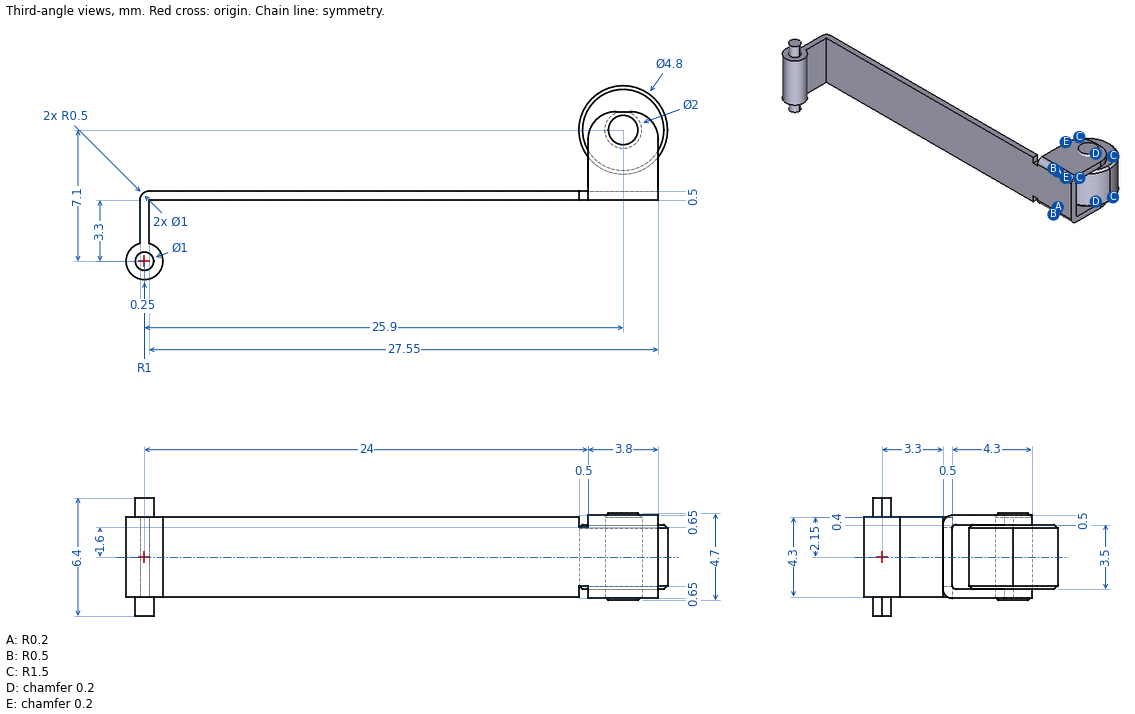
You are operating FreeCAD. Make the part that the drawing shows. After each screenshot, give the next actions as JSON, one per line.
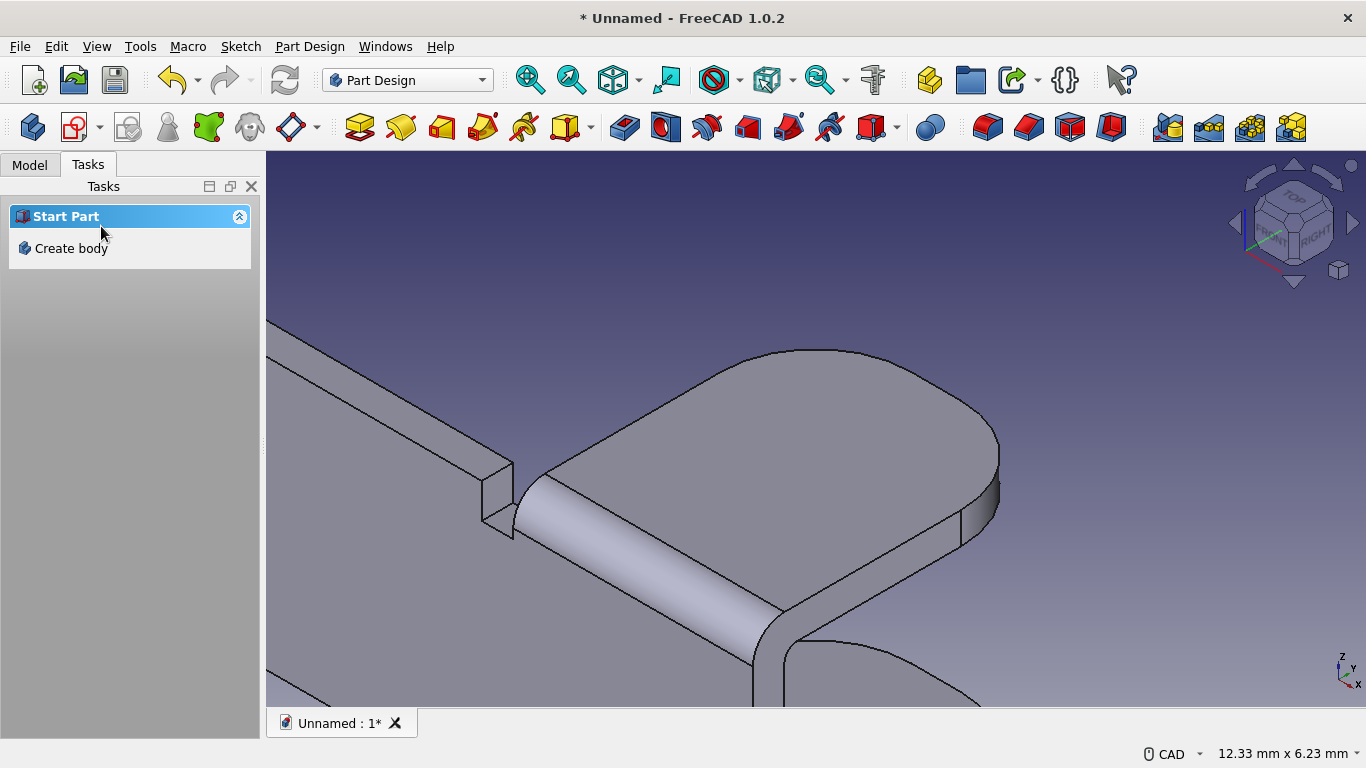
{"action": "left_click", "coordinate": [531, 80]}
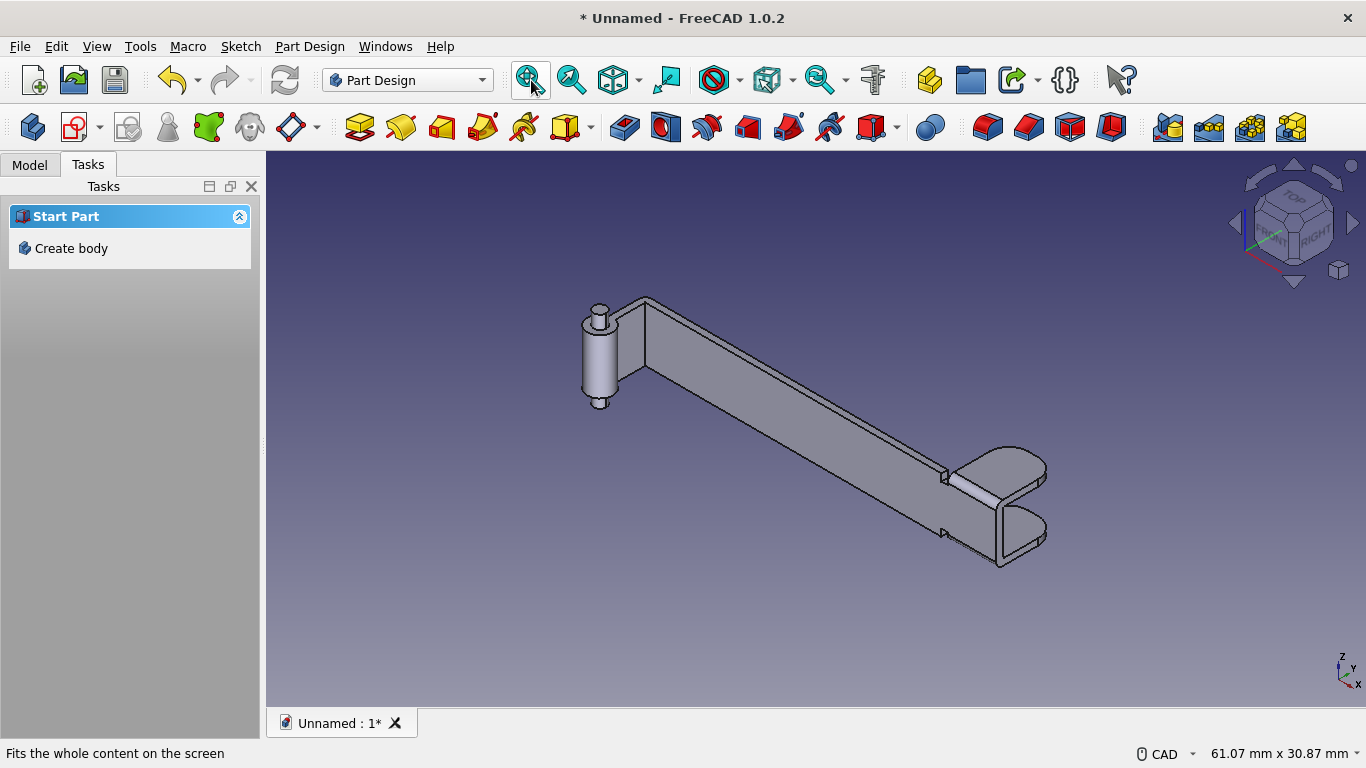
{"action": "left_click", "coordinate": [33, 128]}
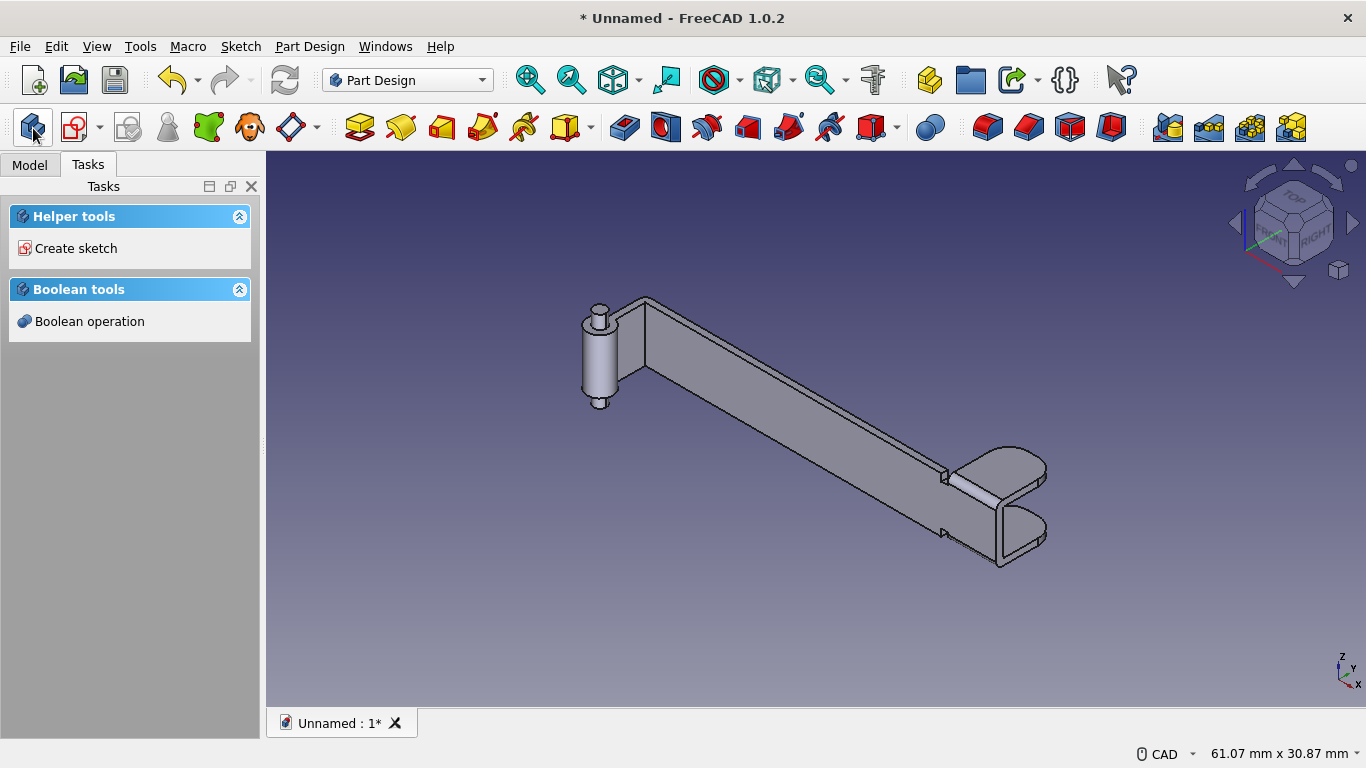
{"action": "left_click", "coordinate": [306, 667]}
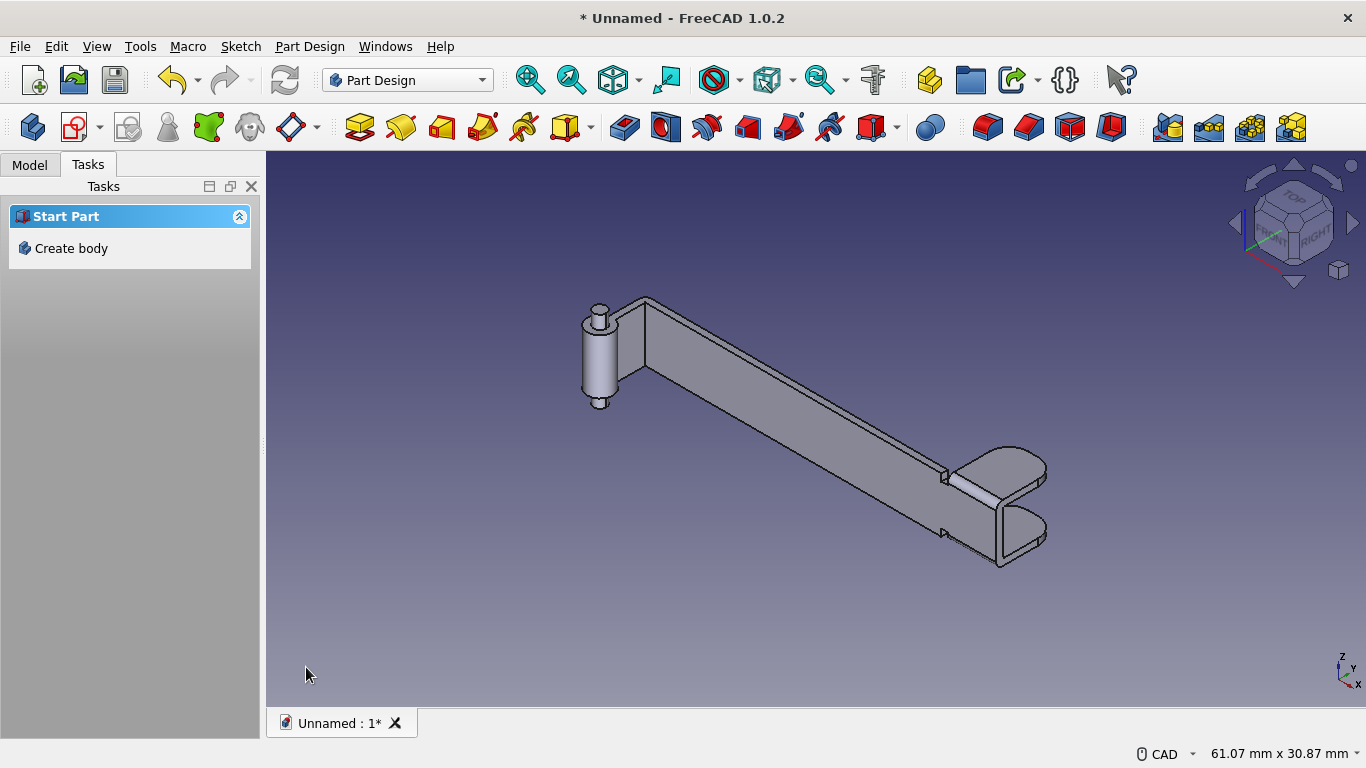
{"action": "left_click", "coordinate": [74, 128]}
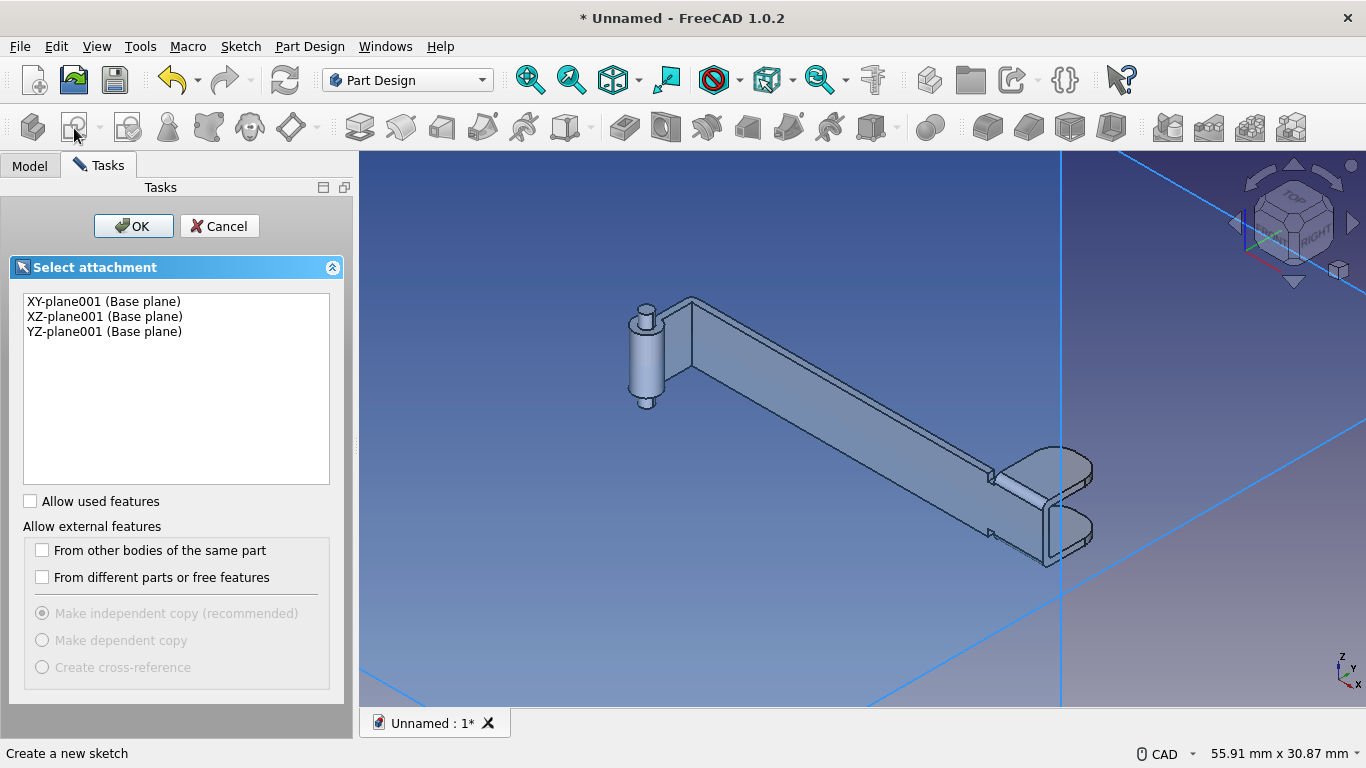
{"action": "left_click", "coordinate": [84, 302]}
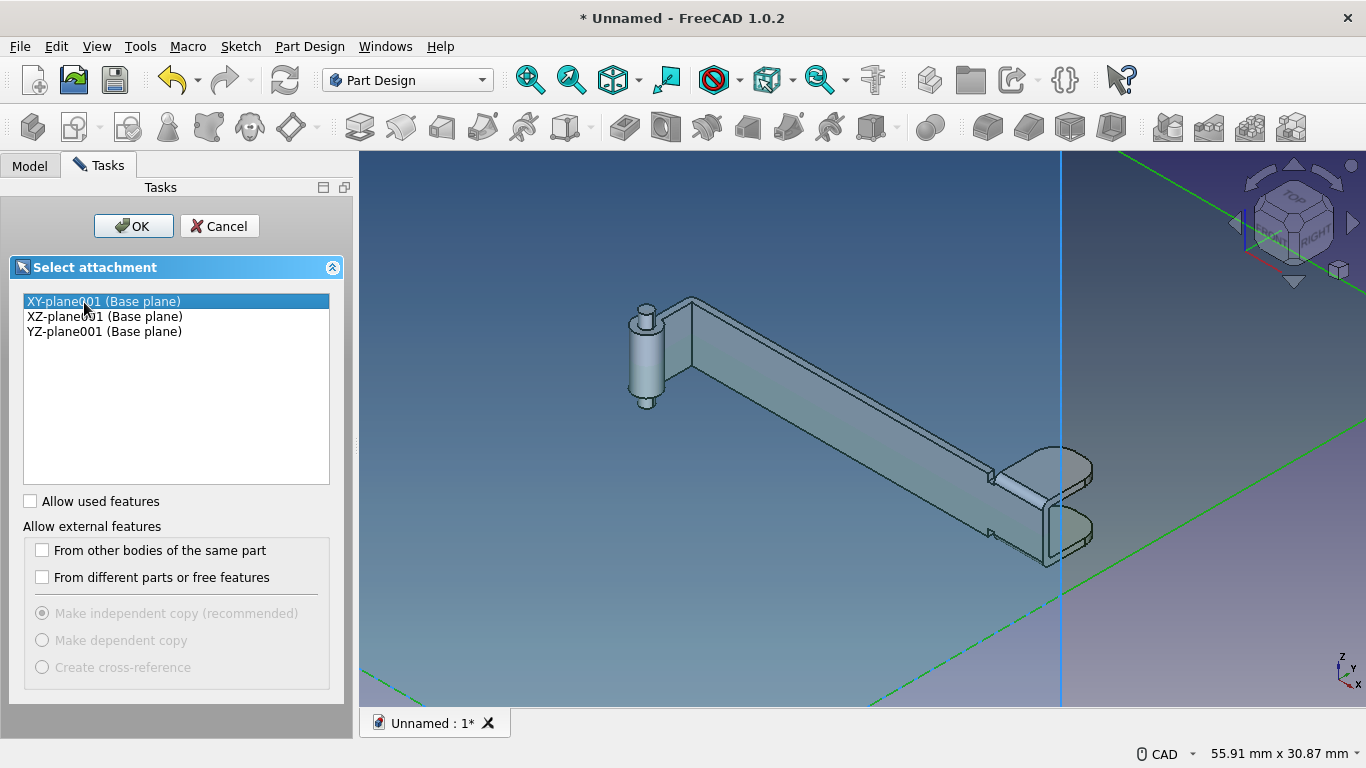
{"action": "left_click", "coordinate": [134, 226]}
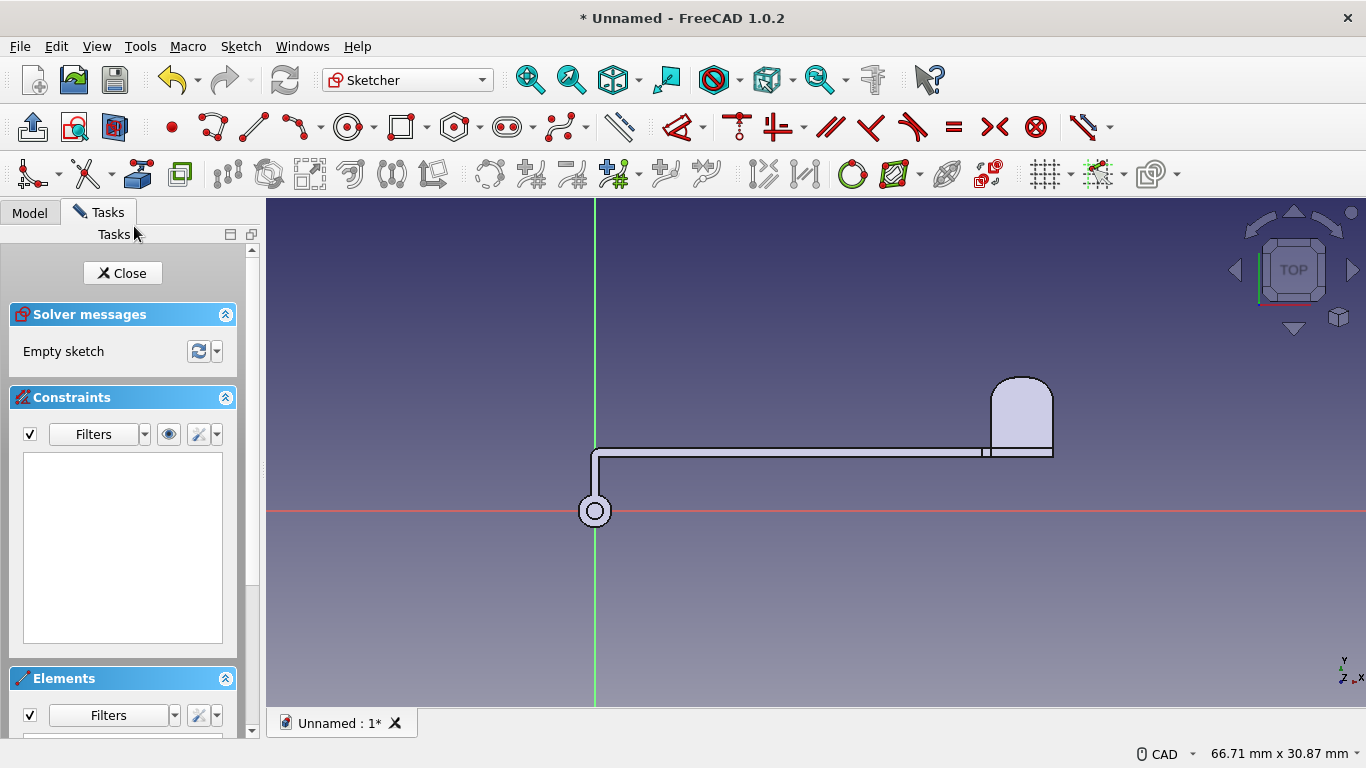
{"action": "scroll", "coordinate": [1056, 387], "scroll_direction": "up", "scroll_amount": 11}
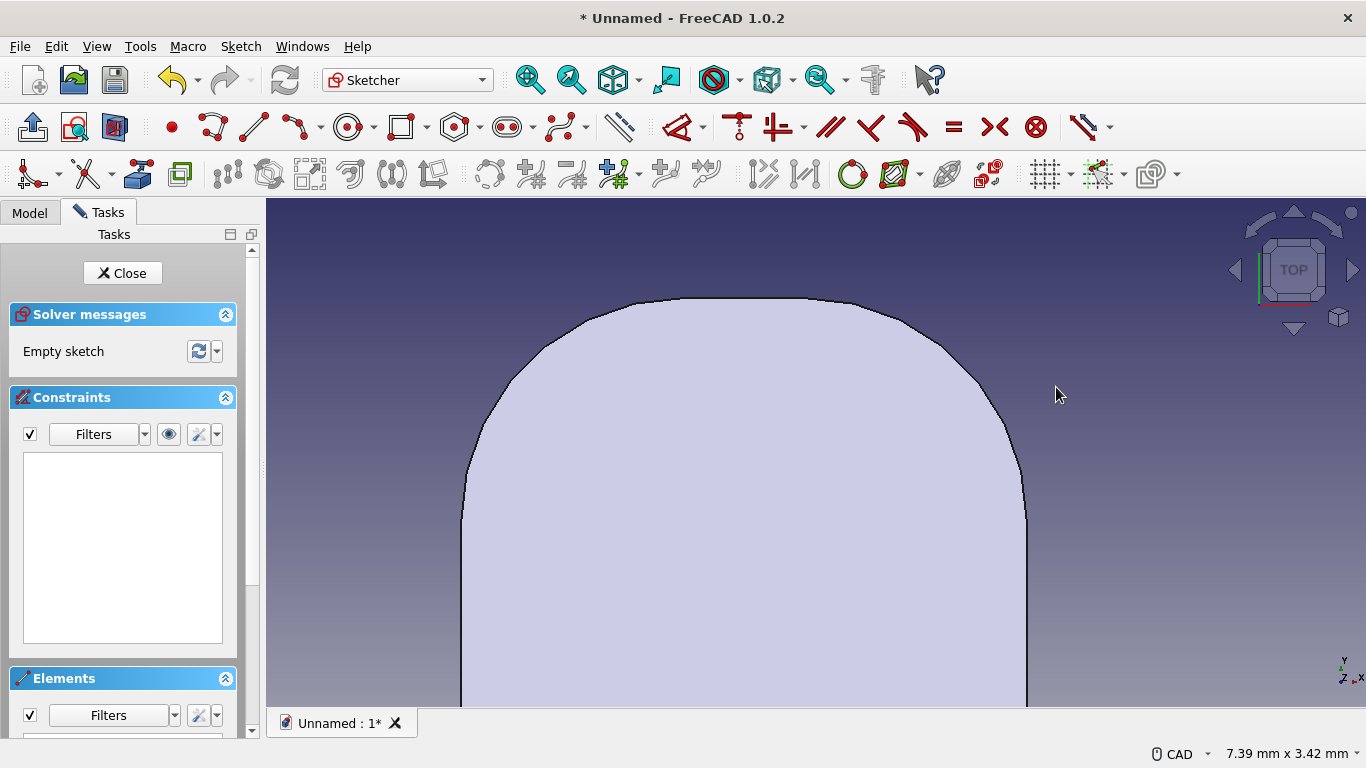
{"action": "left_click", "coordinate": [348, 128]}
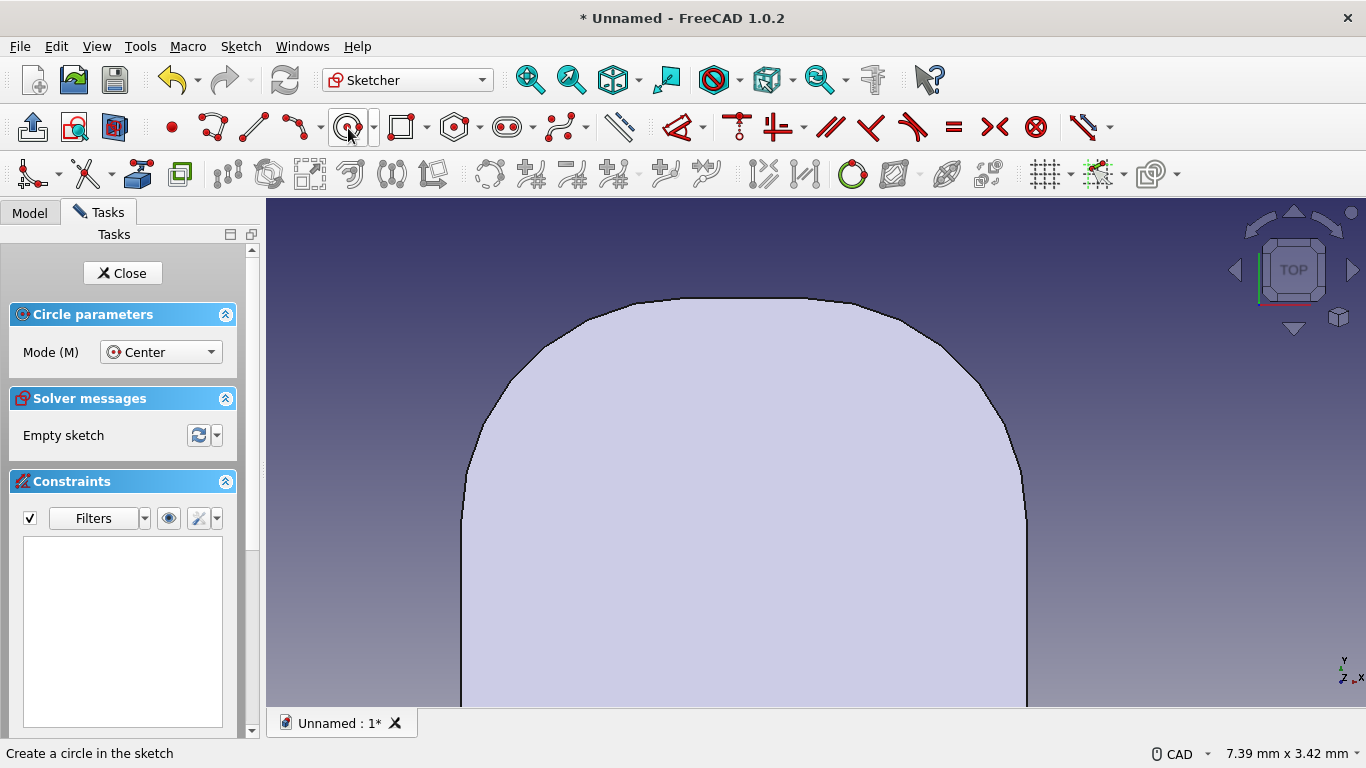
{"action": "left_click", "coordinate": [744, 447]}
{"action": "mouse_move", "coordinate": [849, 342]}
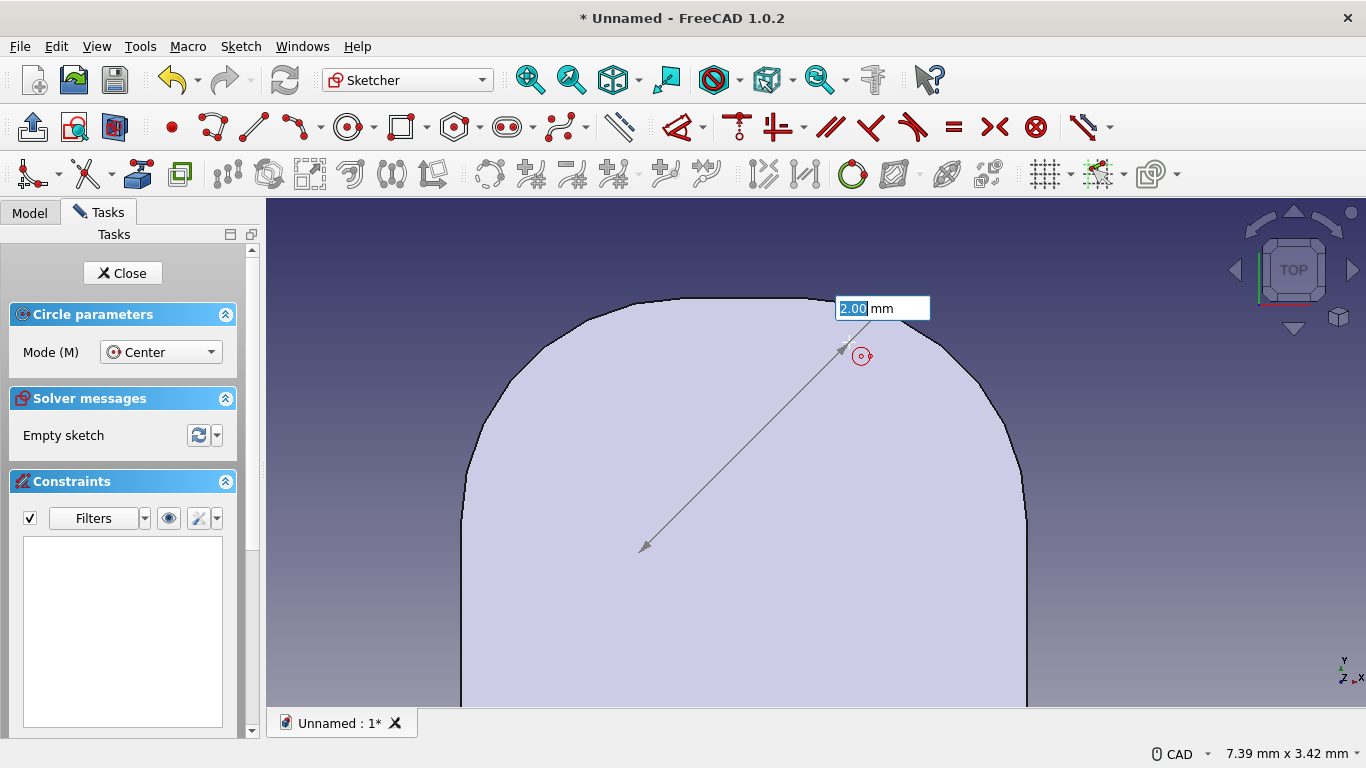
{"action": "type", "text": "2"}
{"action": "key", "text": "Return"}
{"action": "key", "text": "Escape"}